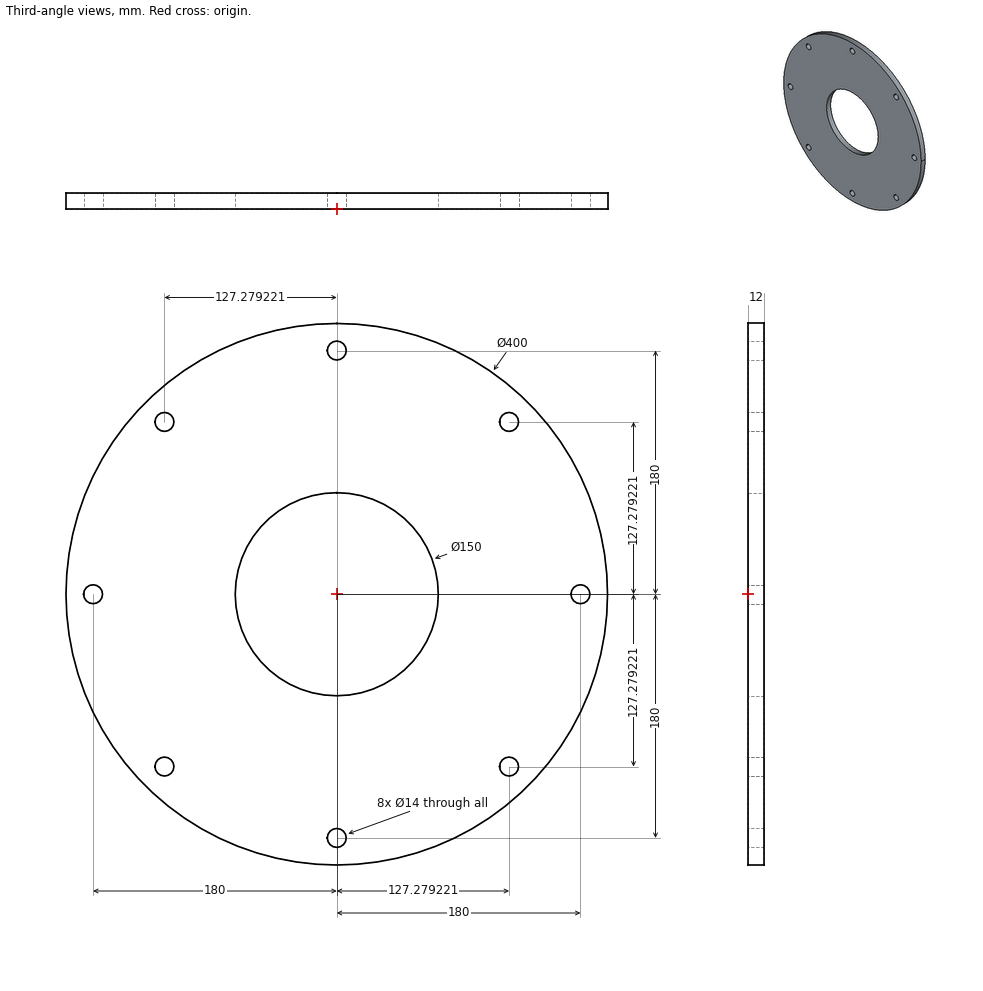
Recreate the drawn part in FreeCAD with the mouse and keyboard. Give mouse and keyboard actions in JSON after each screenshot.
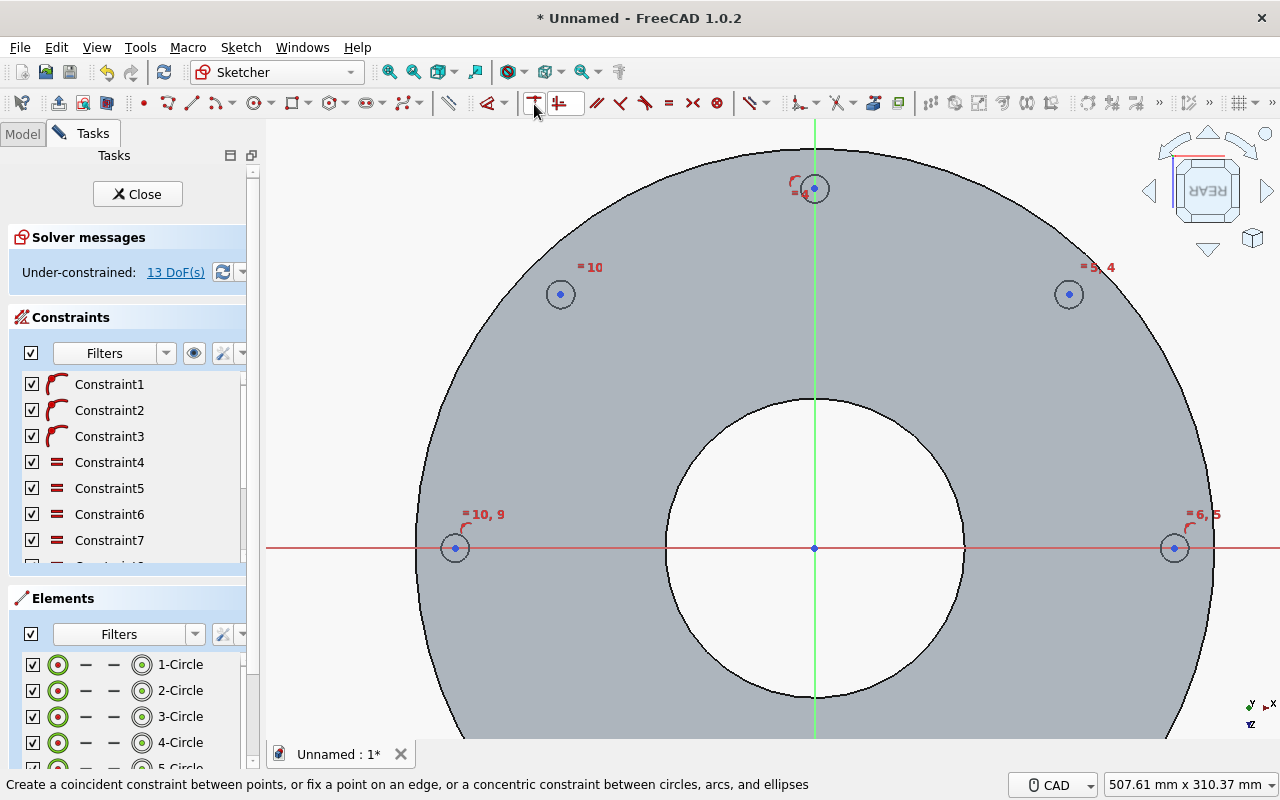
{"action": "left_click", "coordinate": [1069, 295]}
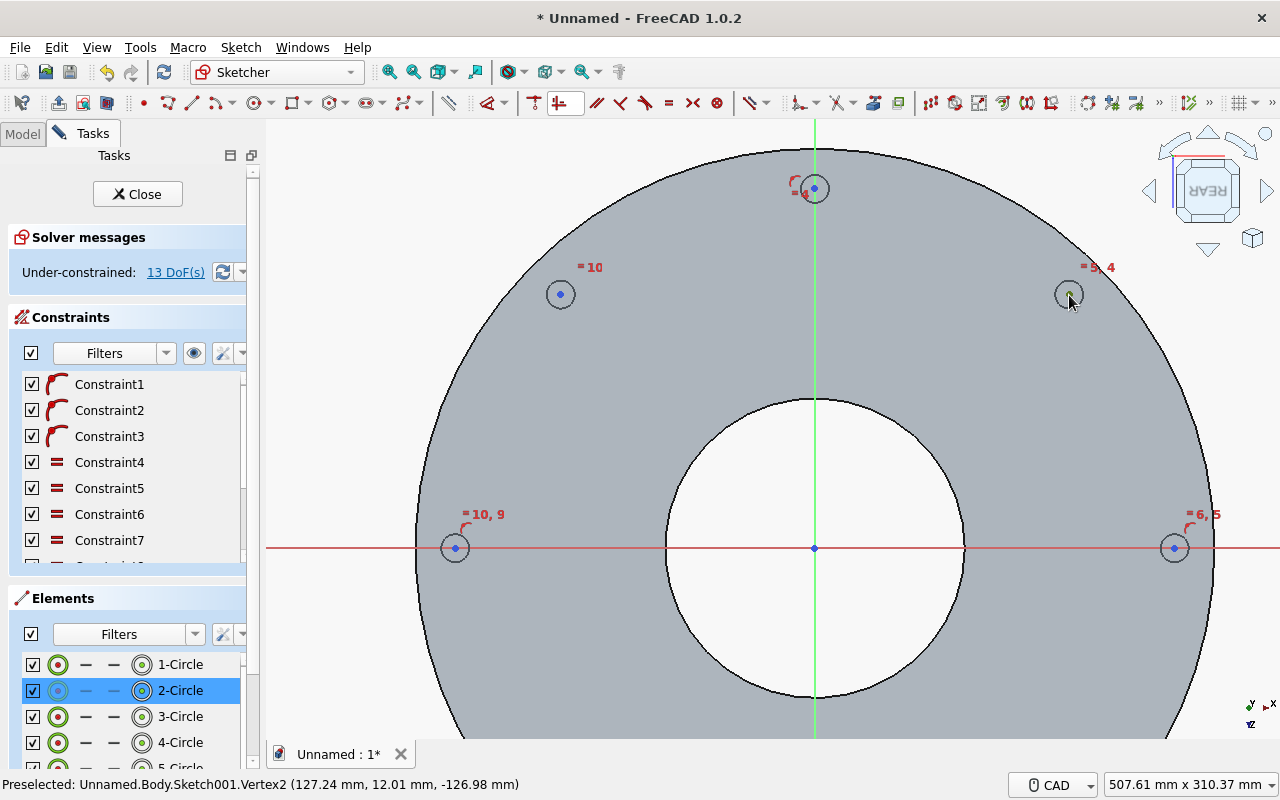
{"action": "scroll", "coordinate": [570, 284], "scroll_direction": "down", "scroll_amount": 3}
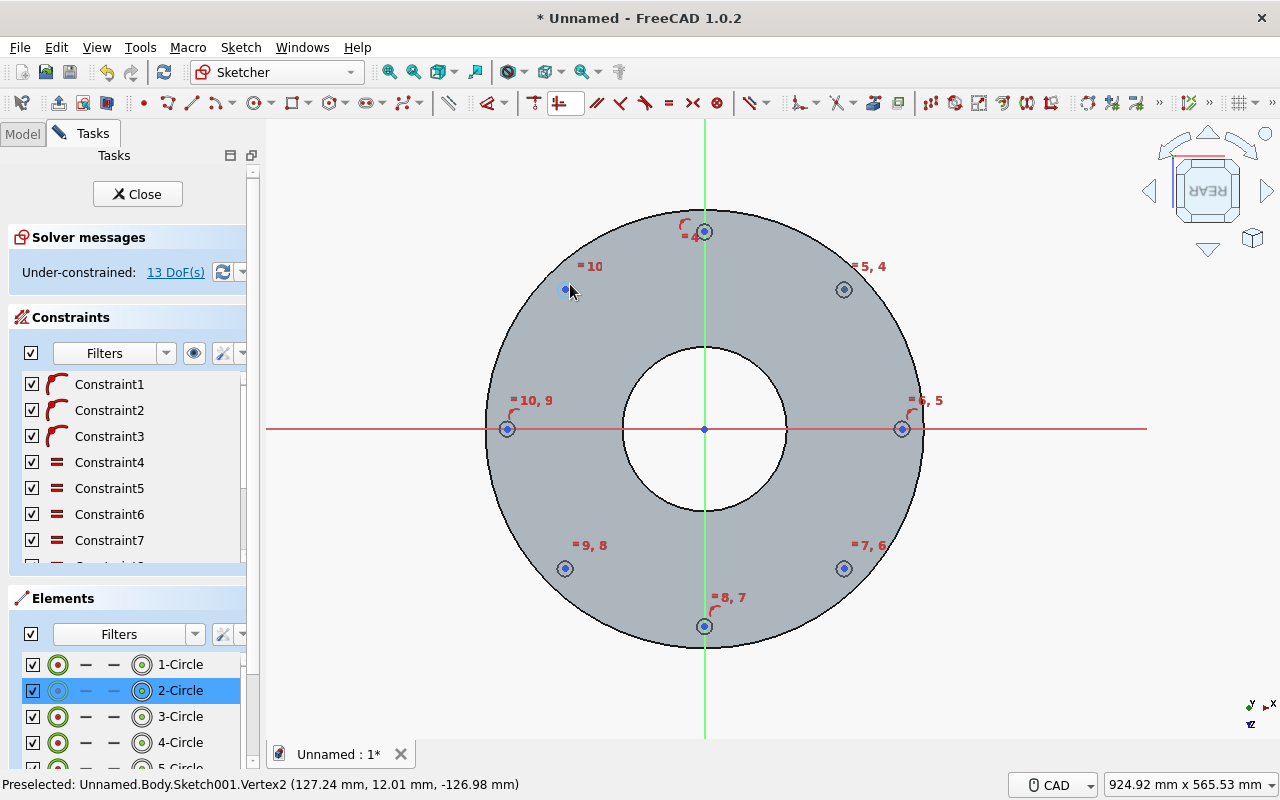
{"action": "left_click", "coordinate": [844, 569]}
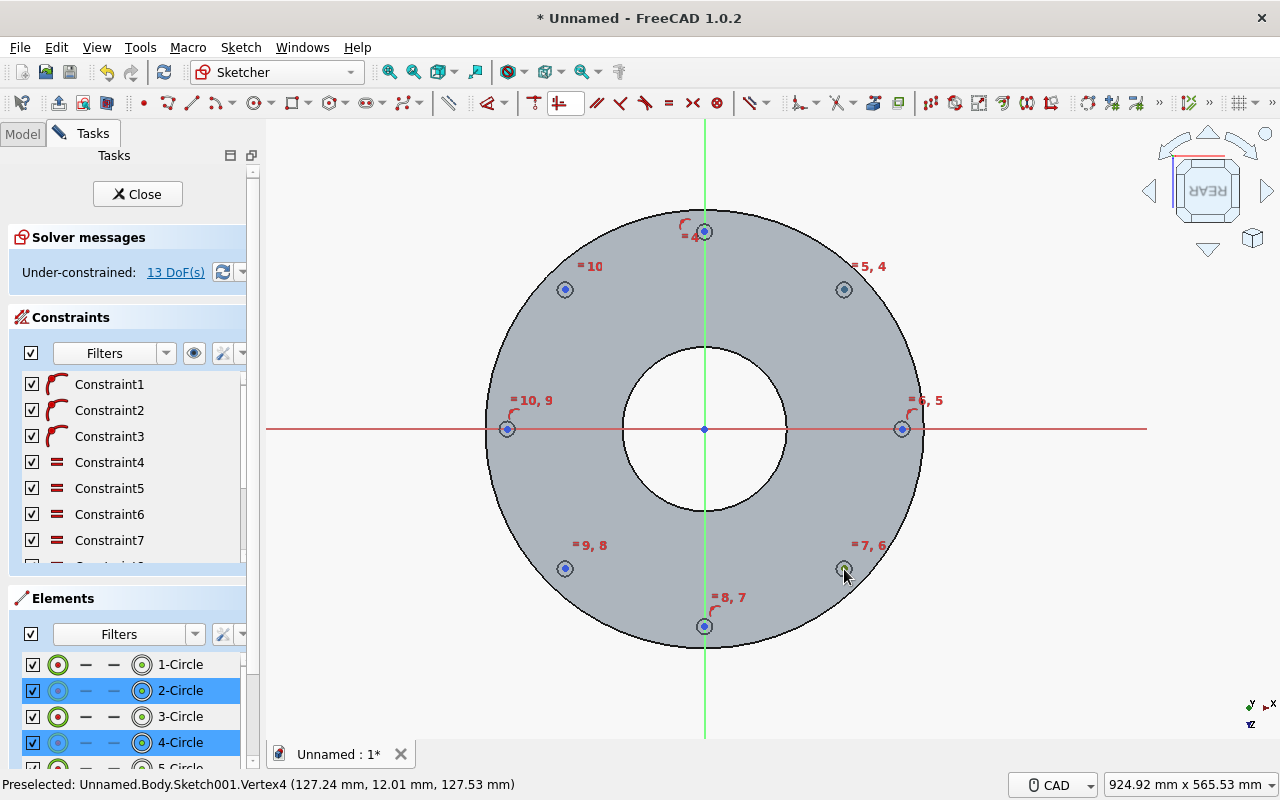
{"action": "left_click", "coordinate": [578, 104]}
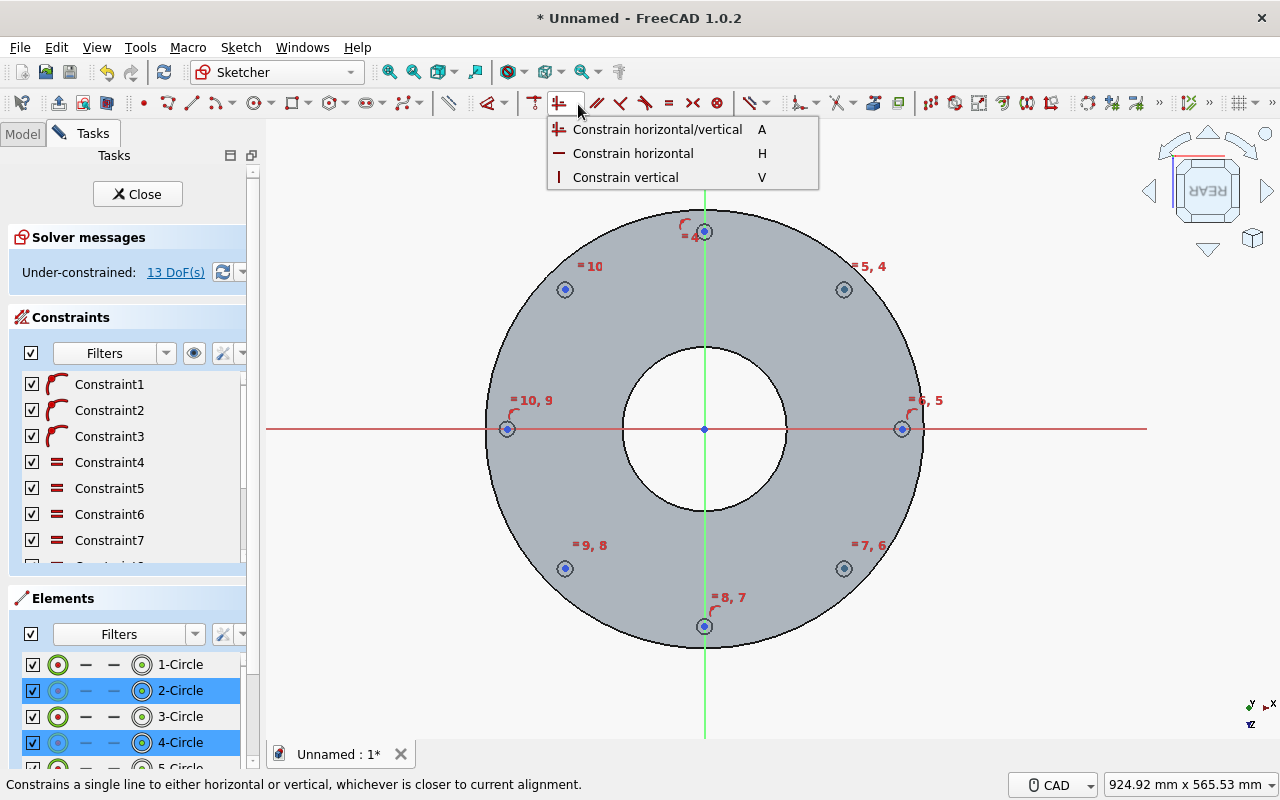
{"action": "left_click", "coordinate": [683, 177]}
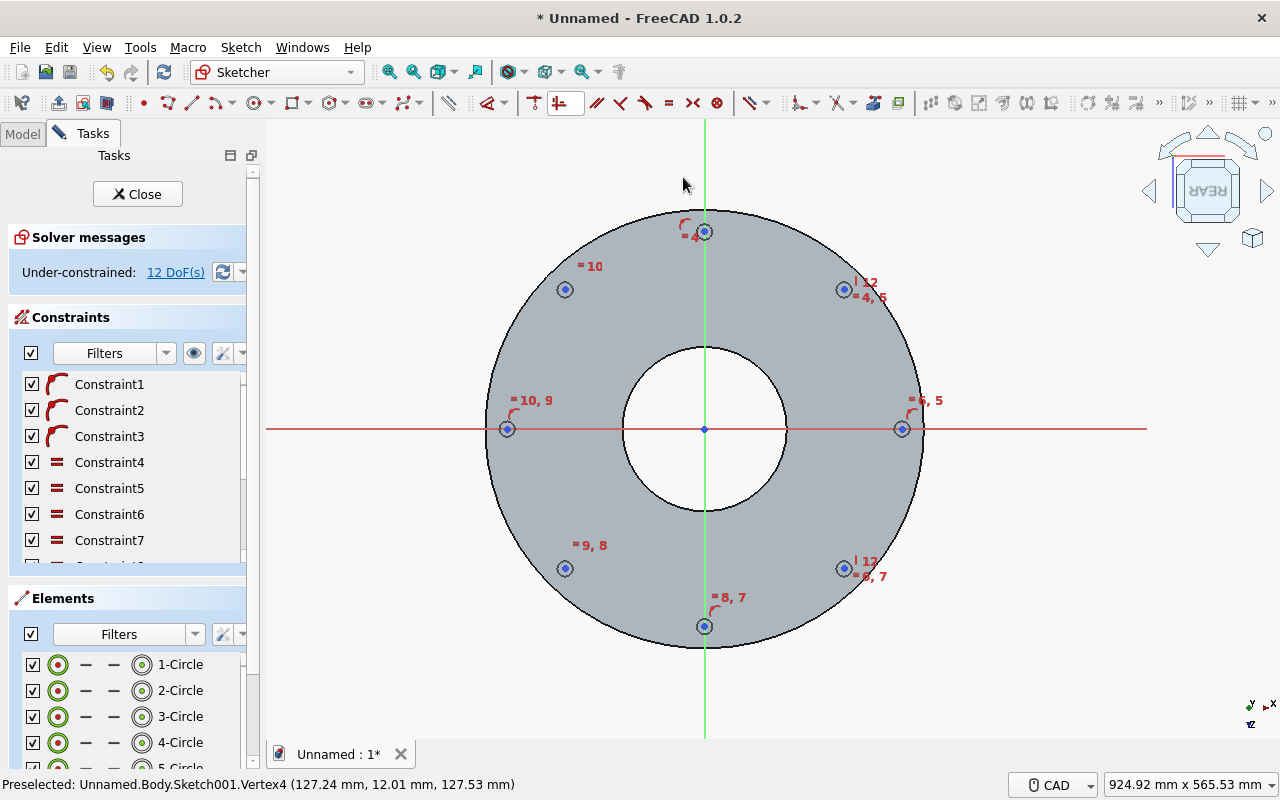
{"action": "left_click", "coordinate": [844, 569]}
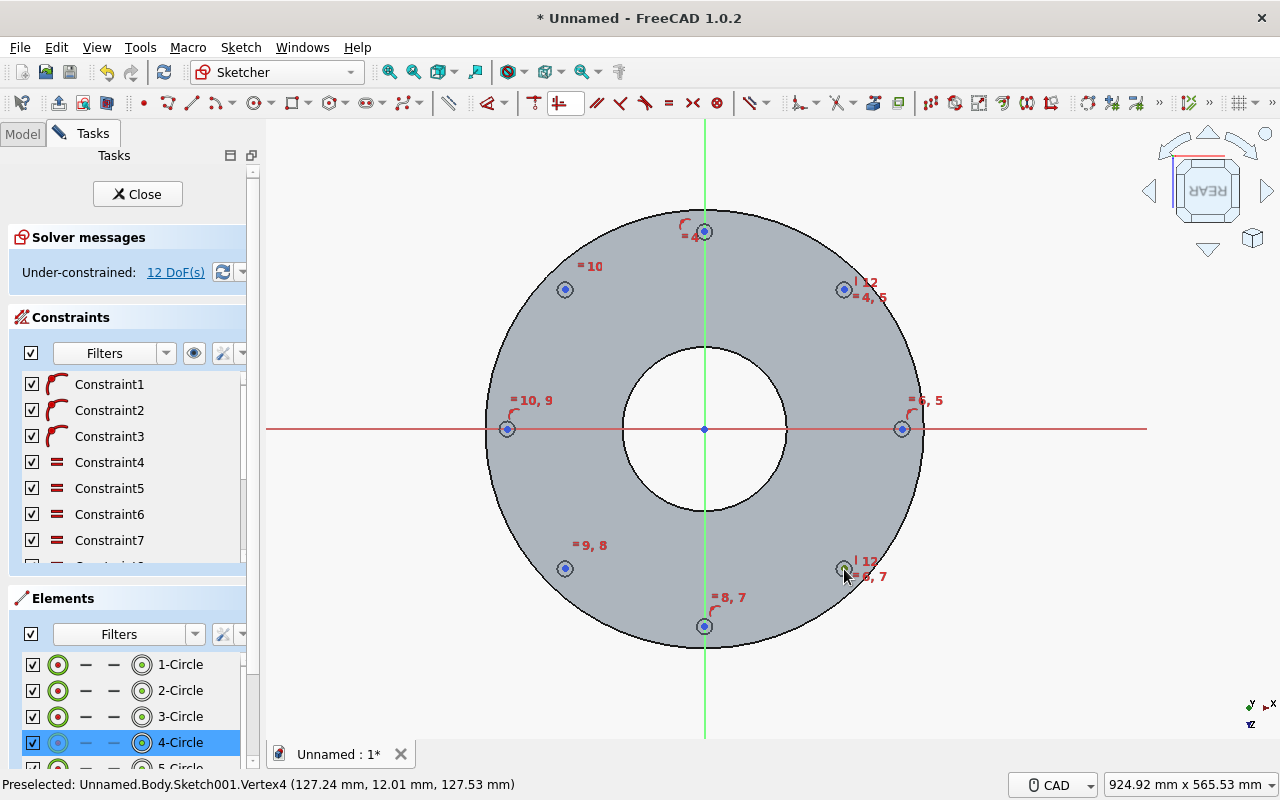
{"action": "left_click", "coordinate": [565, 569]}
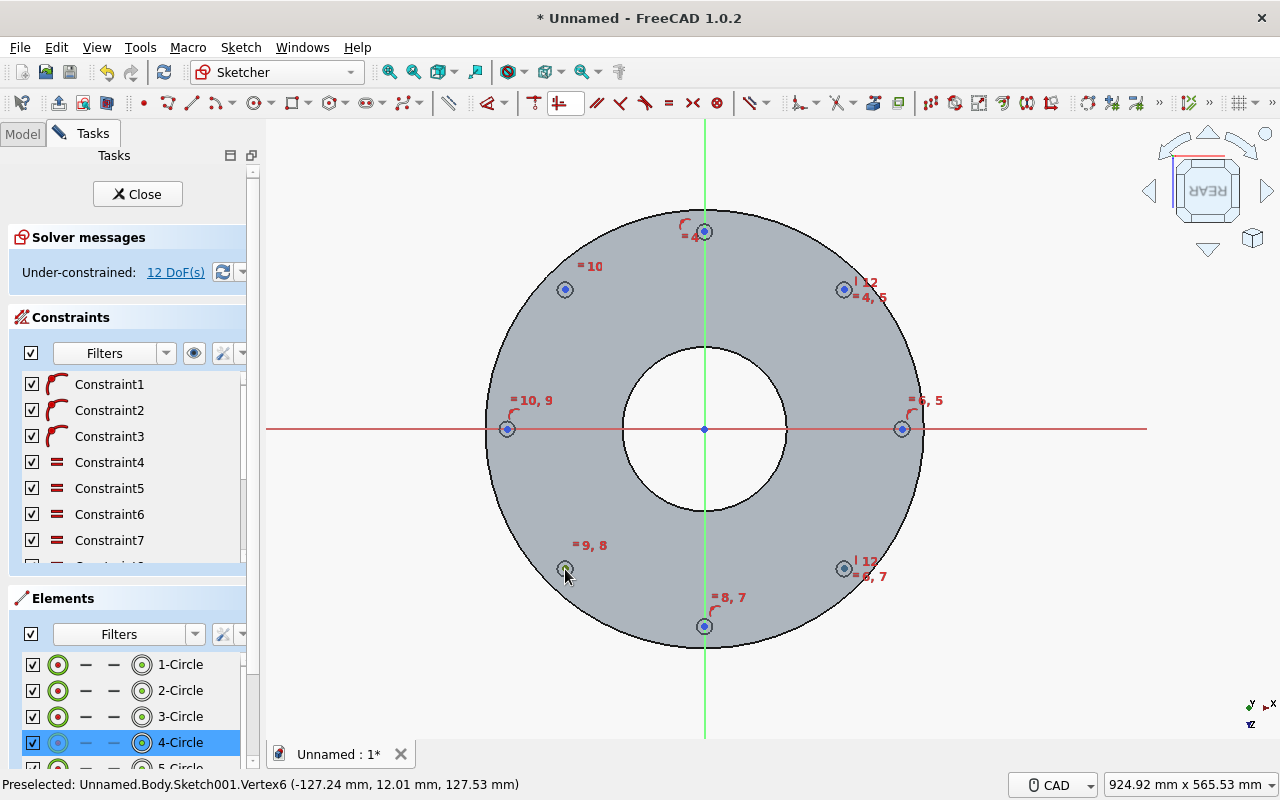
{"action": "left_click", "coordinate": [578, 104]}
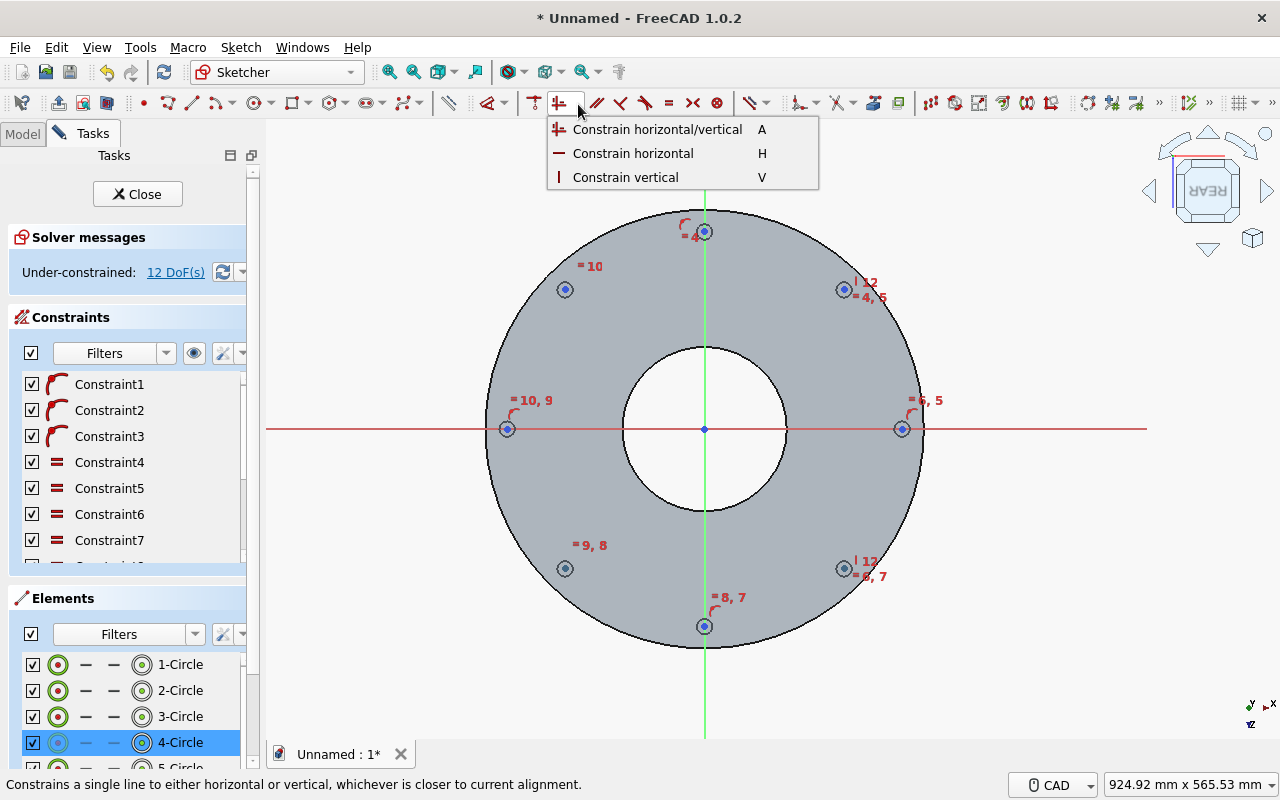
{"action": "left_click", "coordinate": [683, 153]}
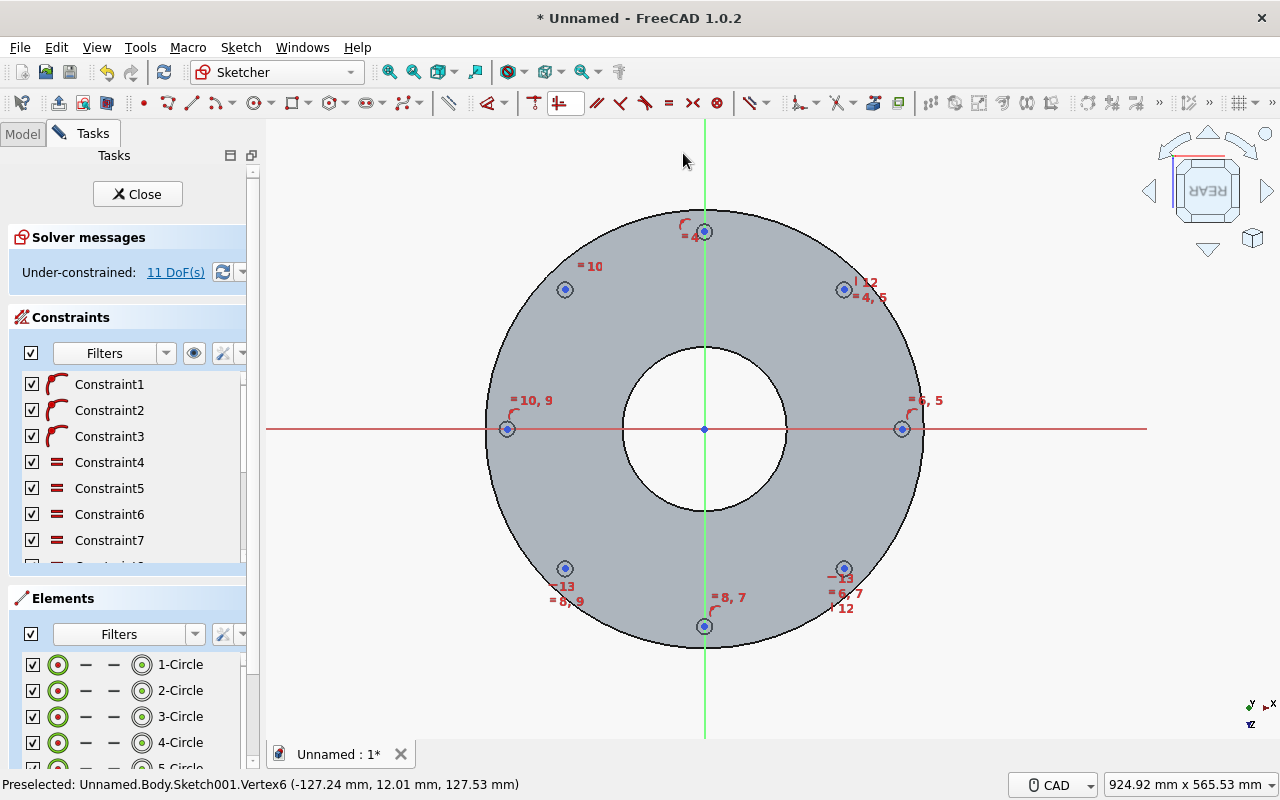
{"action": "left_click", "coordinate": [565, 569]}